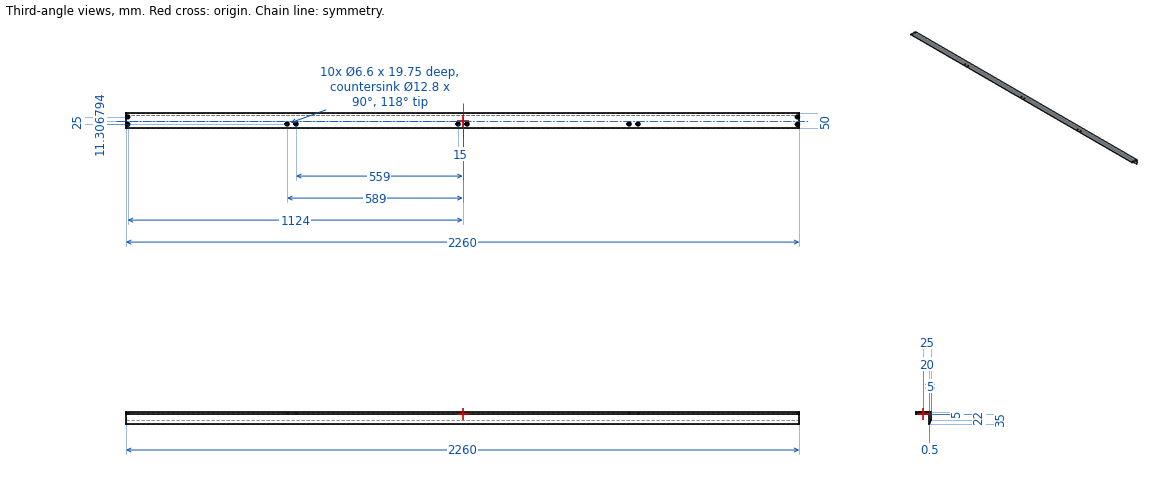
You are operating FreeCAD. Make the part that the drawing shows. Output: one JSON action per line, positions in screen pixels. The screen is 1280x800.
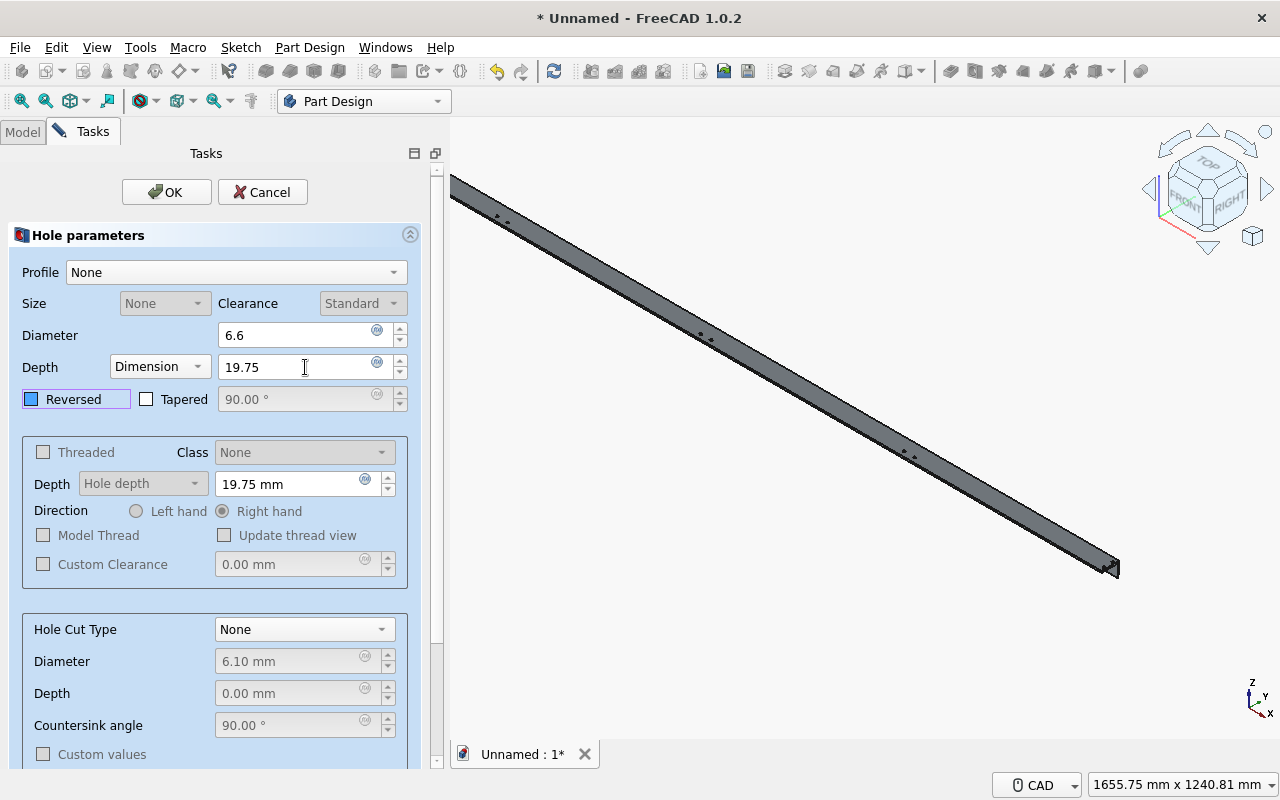
{"action": "left_click", "coordinate": [306, 630]}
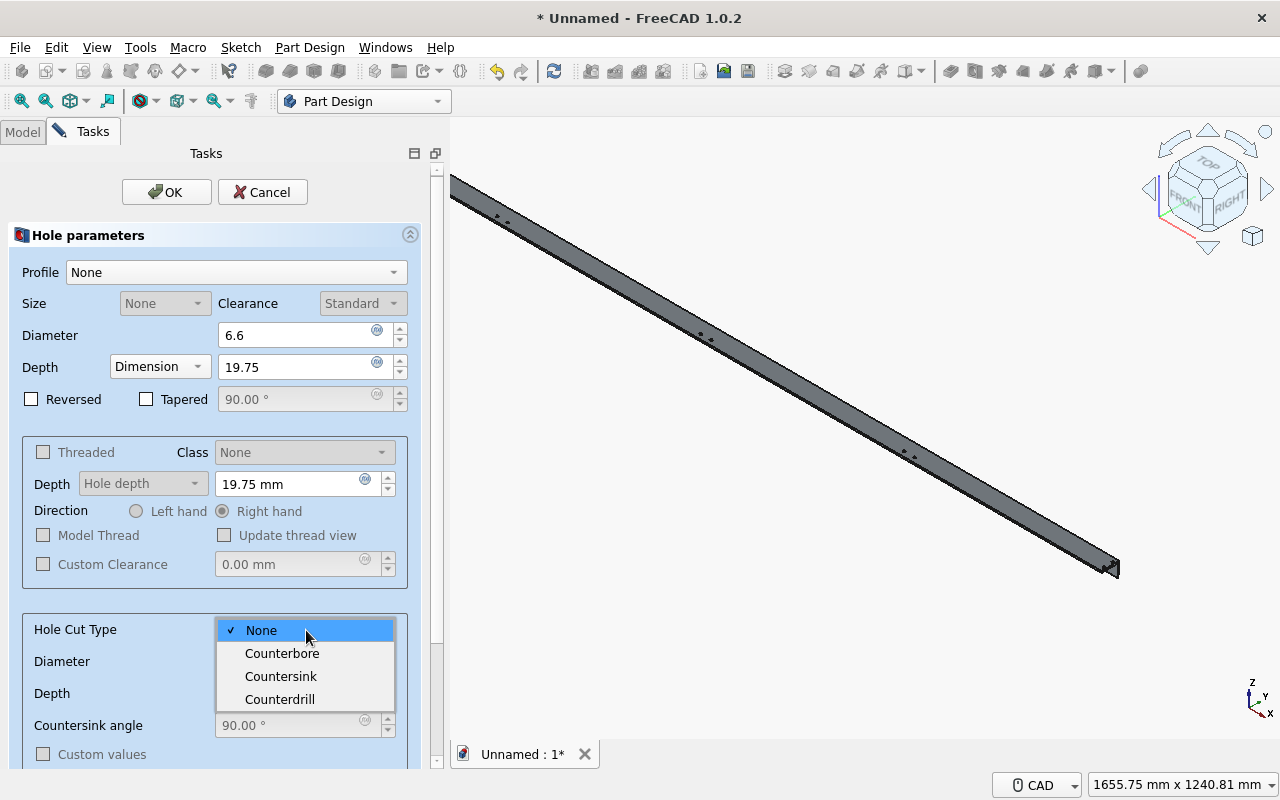
{"action": "left_click", "coordinate": [304, 676]}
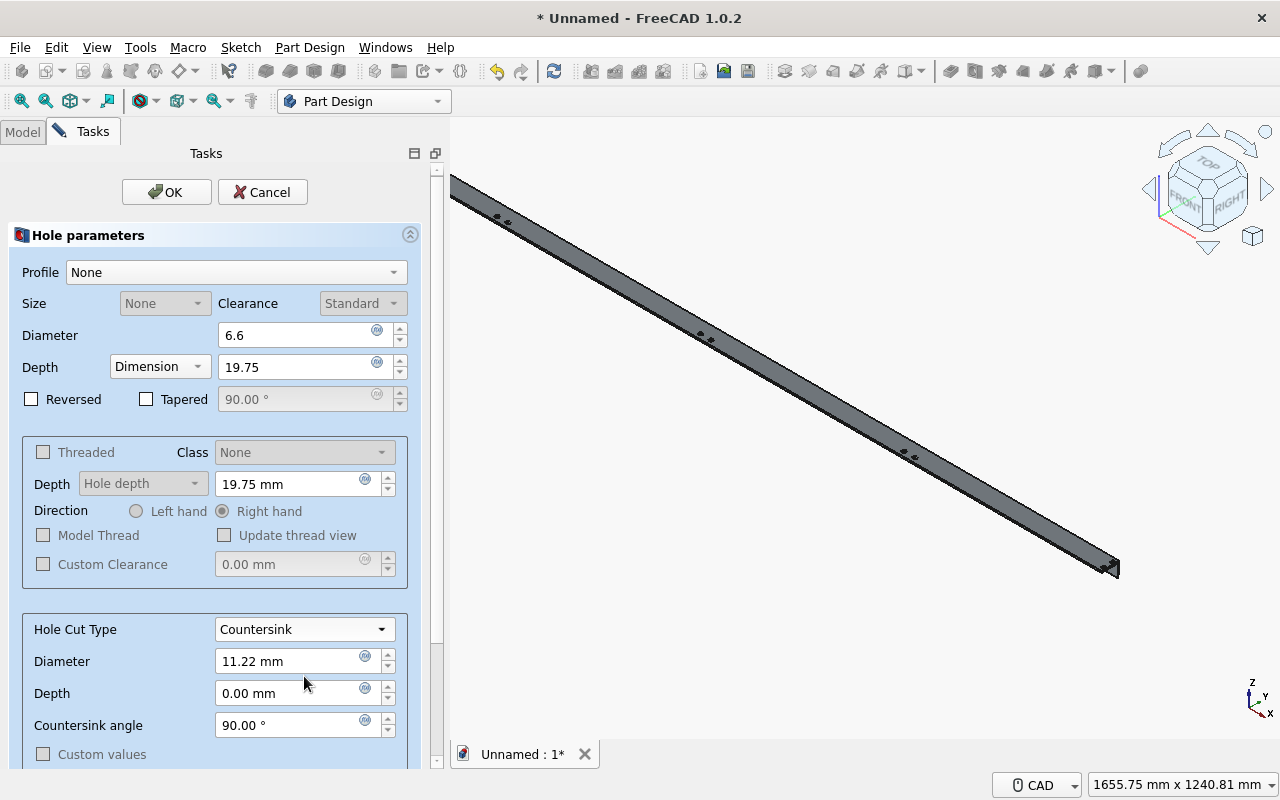
{"action": "triple_click", "coordinate": [298, 661]}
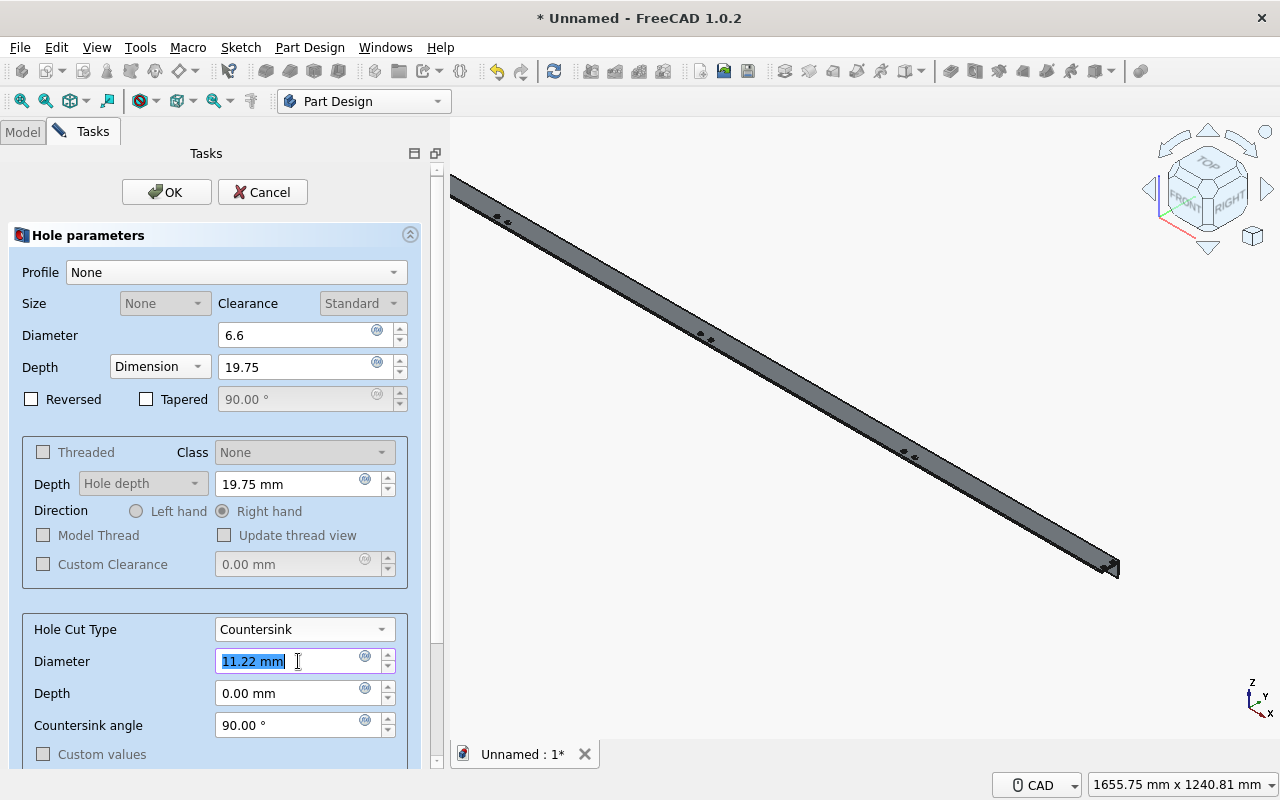
{"action": "type", "text": "12.8"}
{"action": "key", "text": "Tab"}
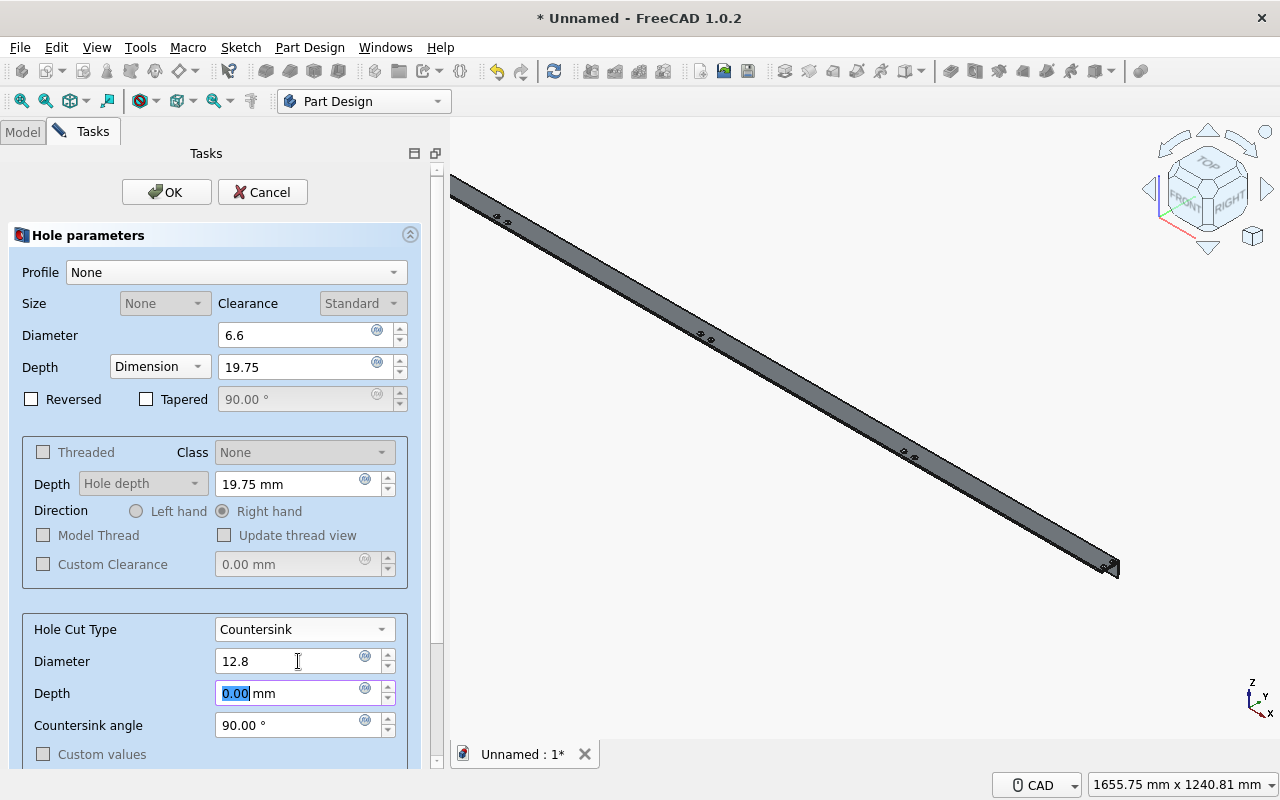
{"action": "left_click", "coordinate": [167, 192]}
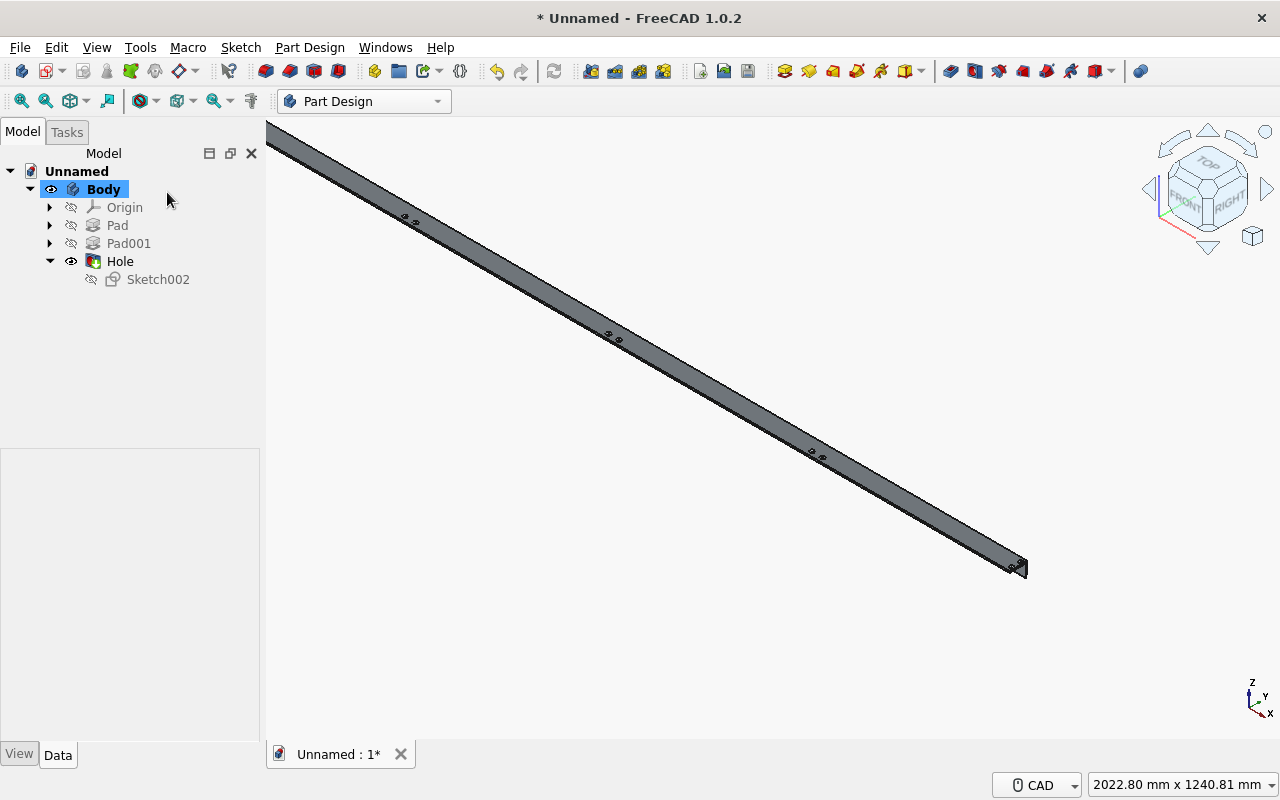
{"action": "left_click", "coordinate": [22, 102]}